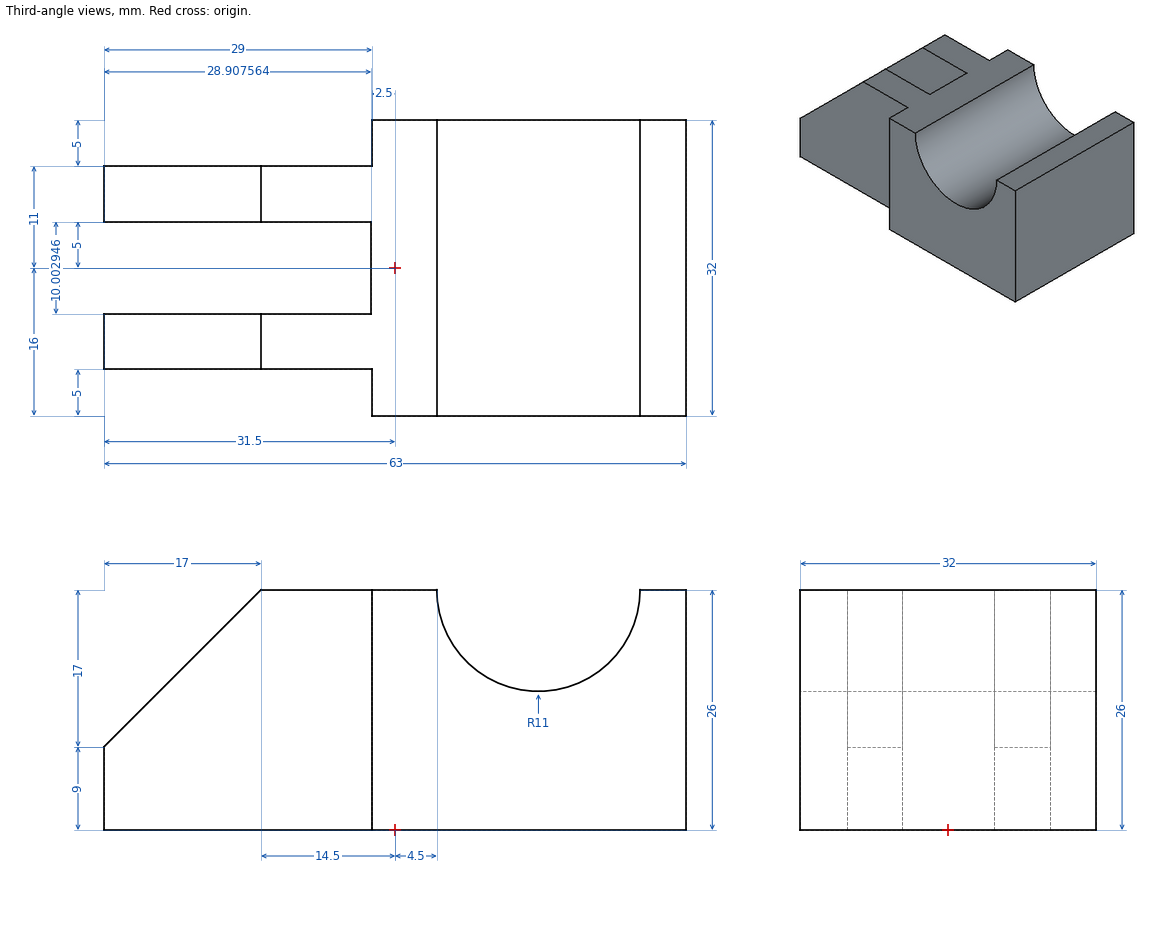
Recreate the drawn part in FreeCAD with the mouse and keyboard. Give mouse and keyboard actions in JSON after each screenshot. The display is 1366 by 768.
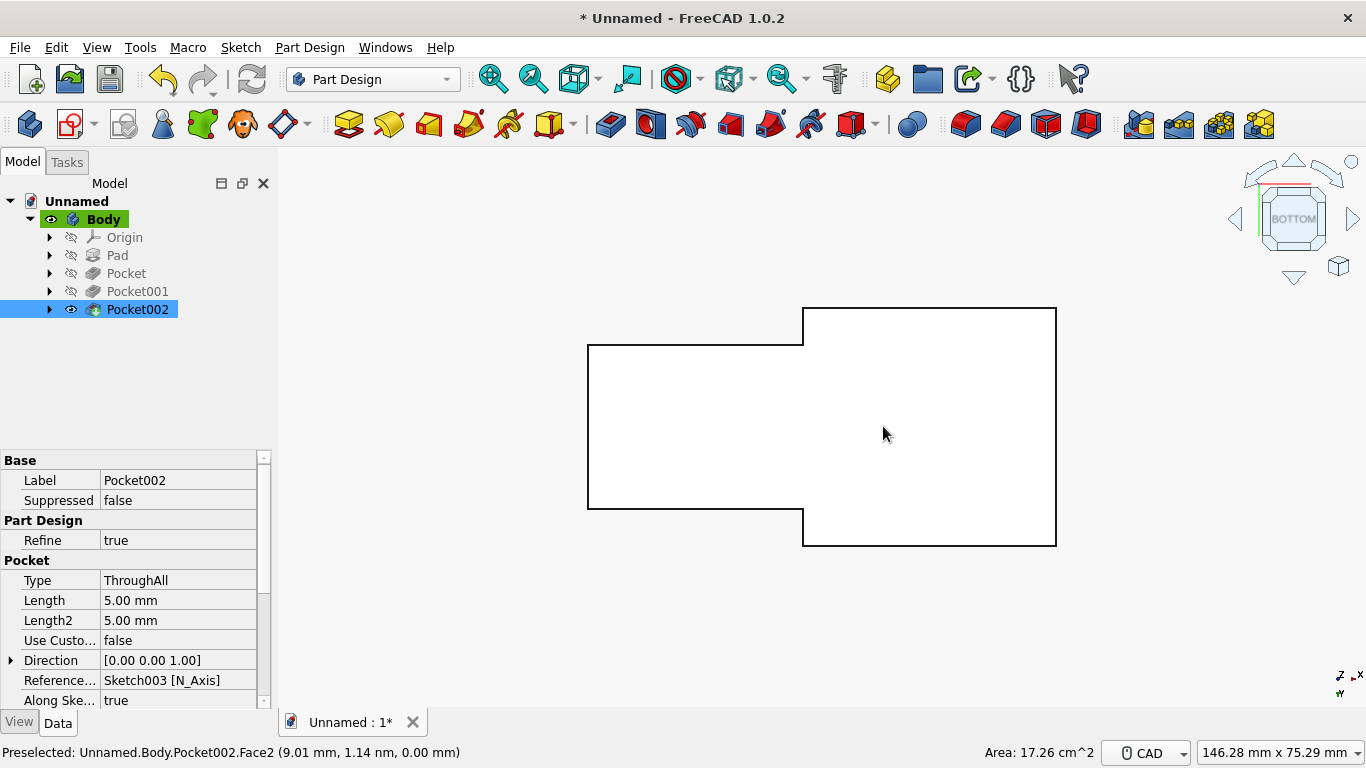
{"action": "left_click", "coordinate": [70, 124]}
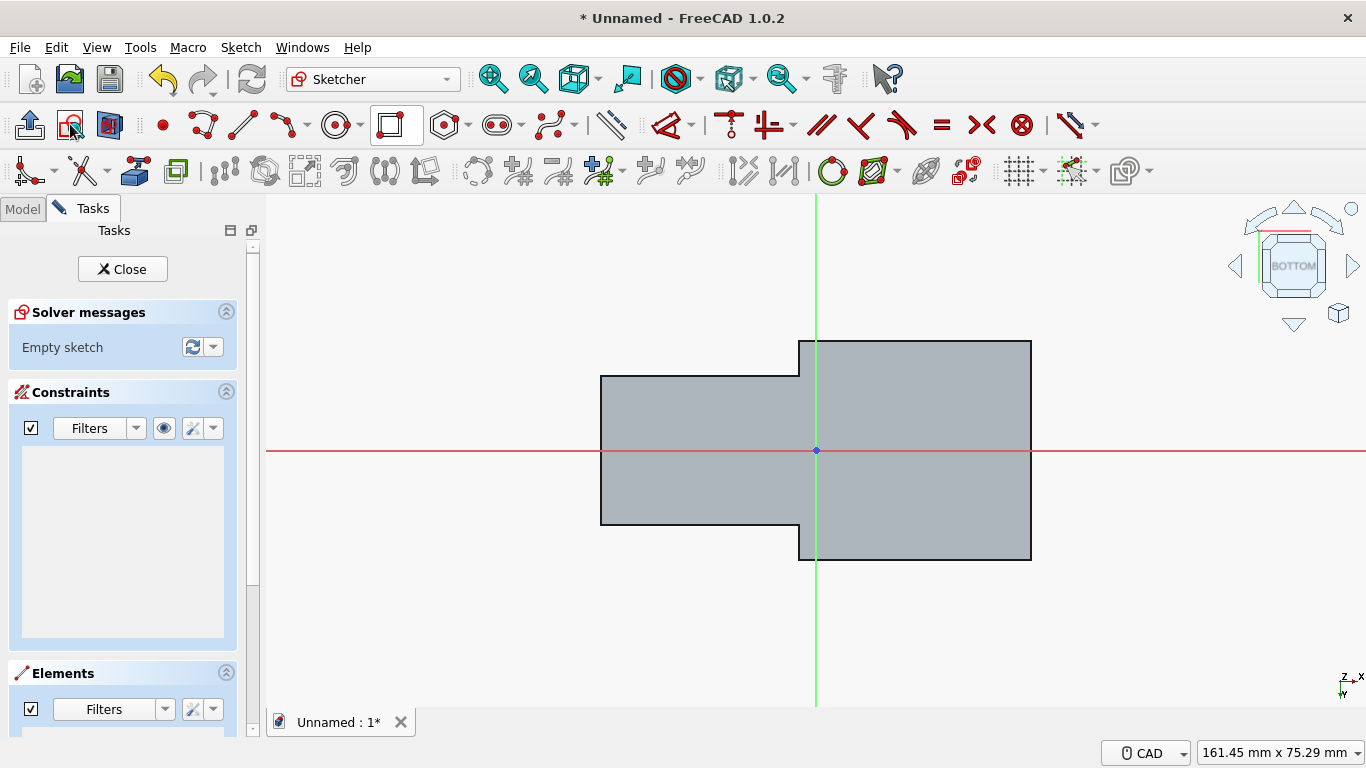
{"action": "scroll", "coordinate": [686, 450], "scroll_direction": "up", "scroll_amount": 5}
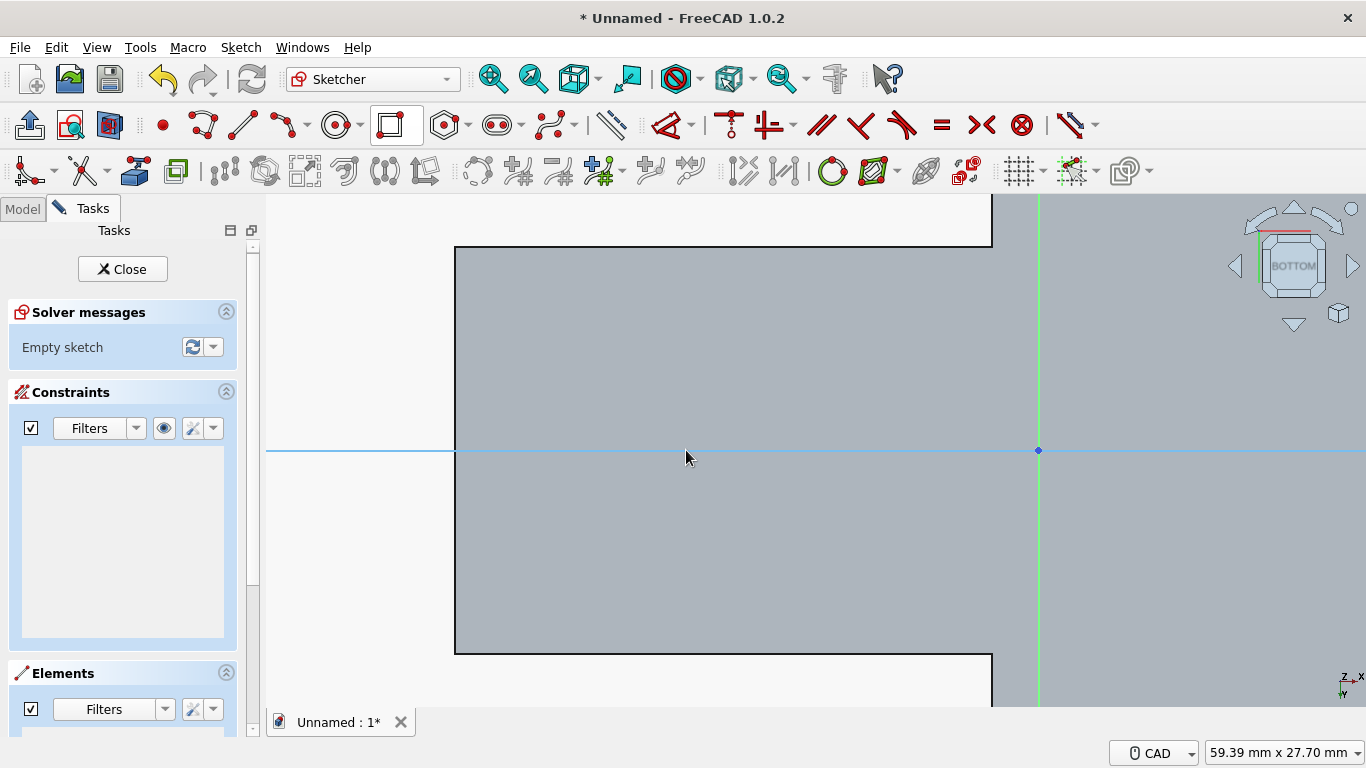
{"action": "left_click", "coordinate": [390, 126]}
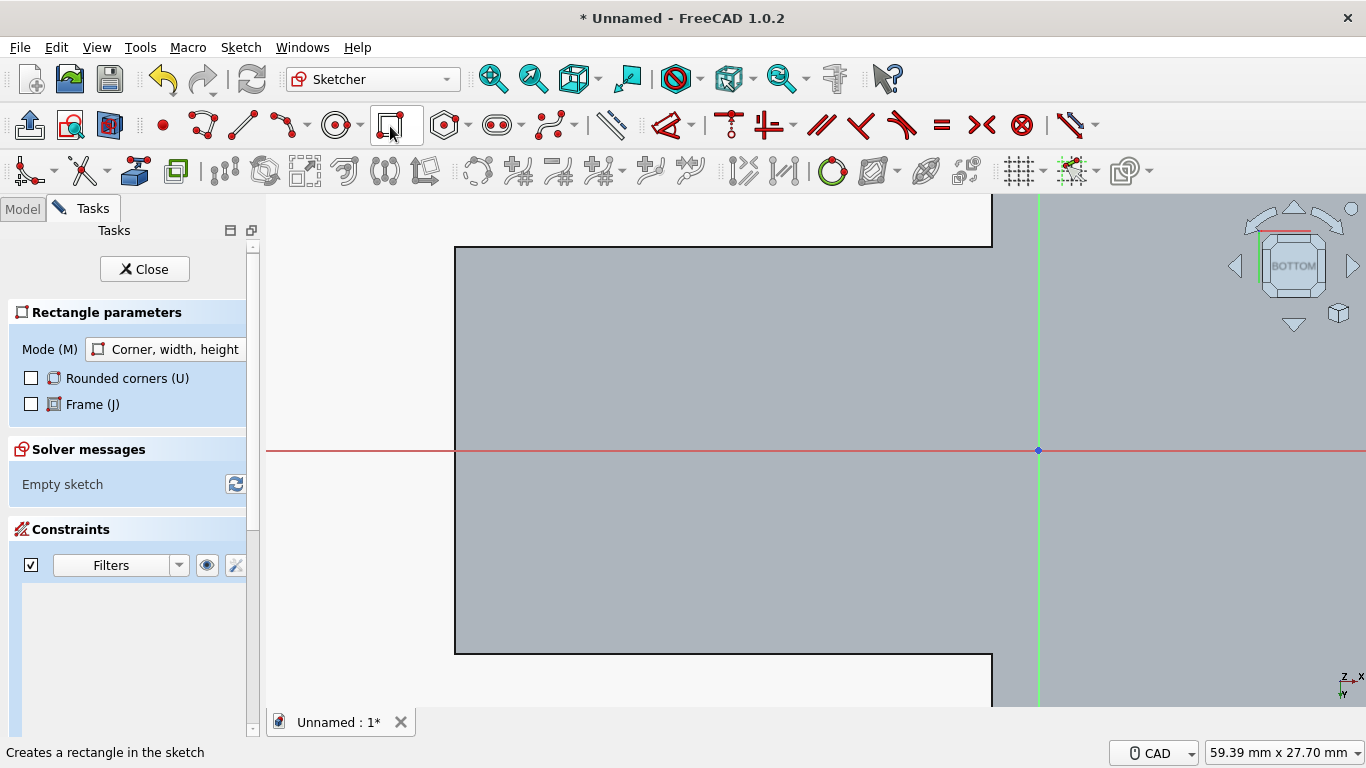
{"action": "left_click", "coordinate": [455, 358]}
{"action": "left_click", "coordinate": [991, 543]}
{"action": "key", "text": "Escape"}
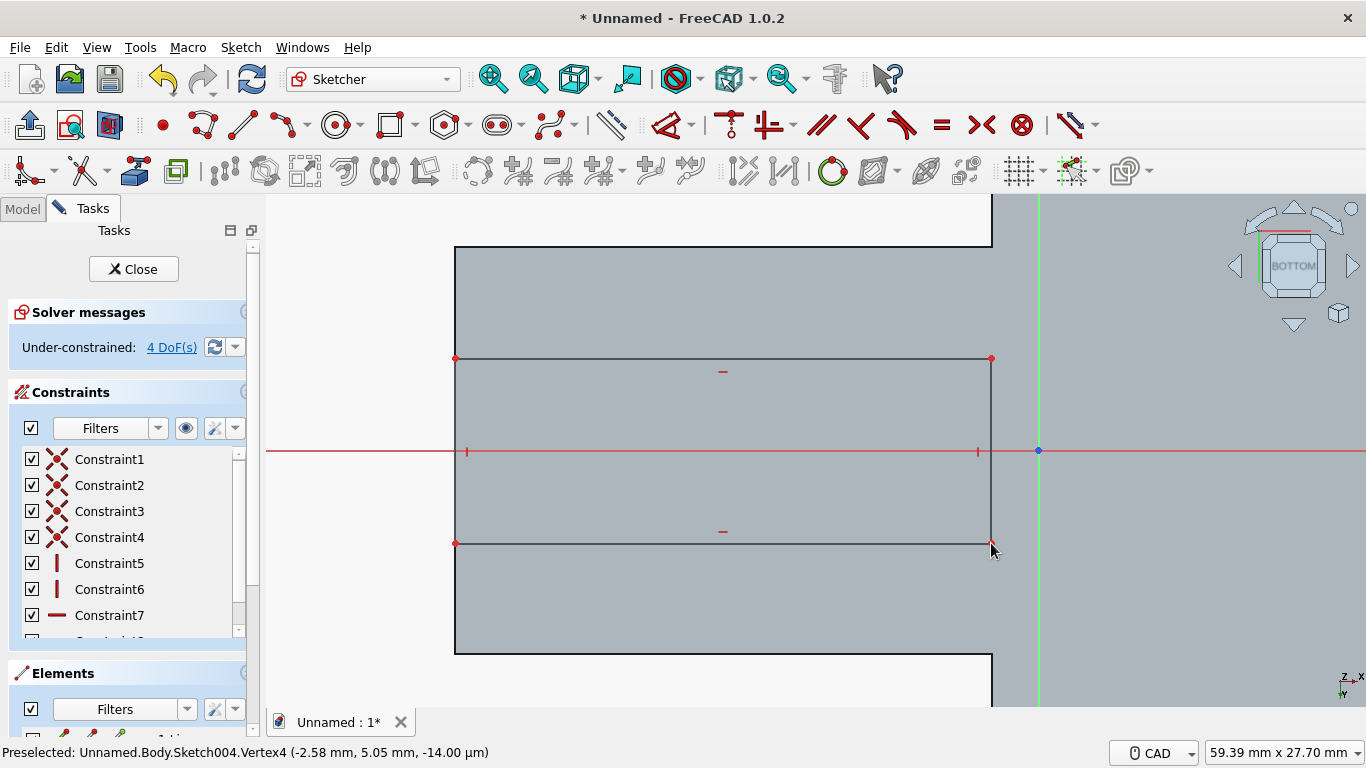
{"action": "left_click", "coordinate": [666, 126]}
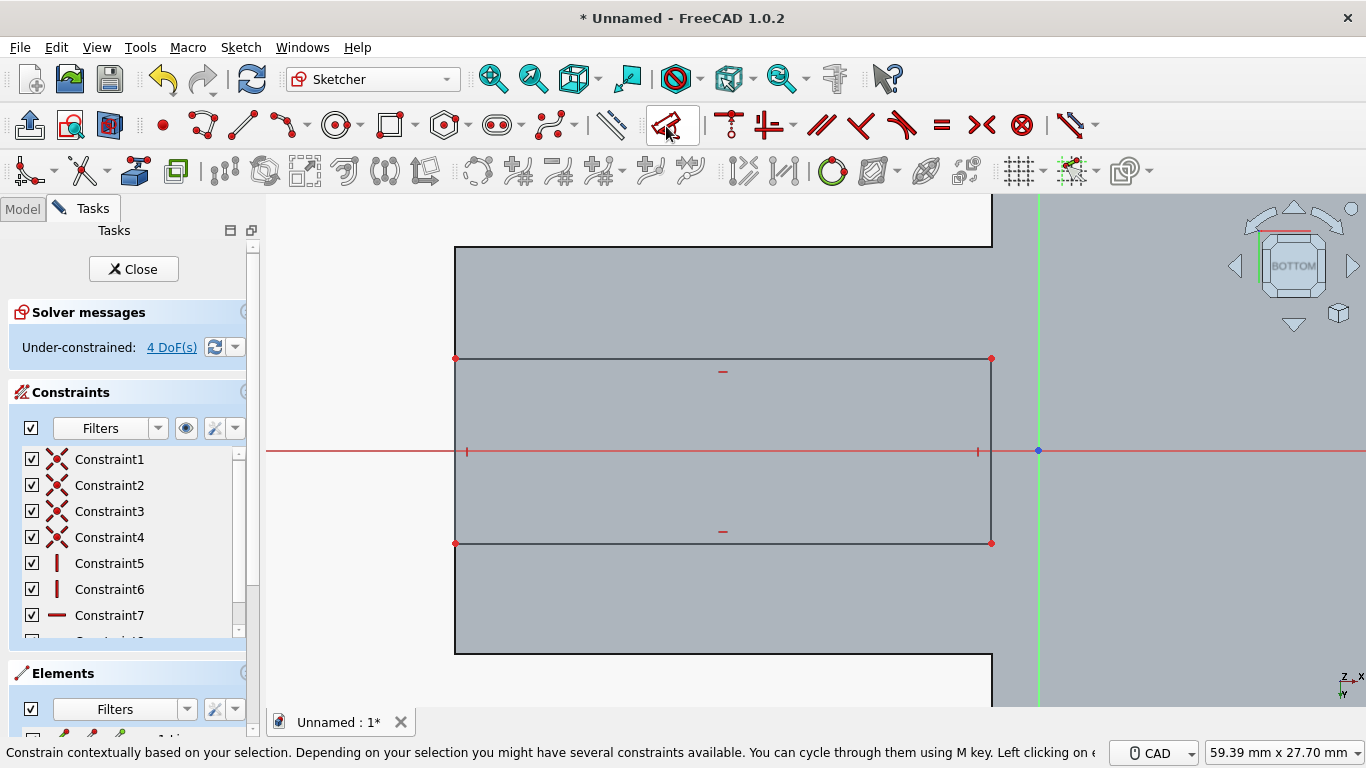
{"action": "left_click", "coordinate": [455, 544]}
{"action": "left_click", "coordinate": [421, 497]}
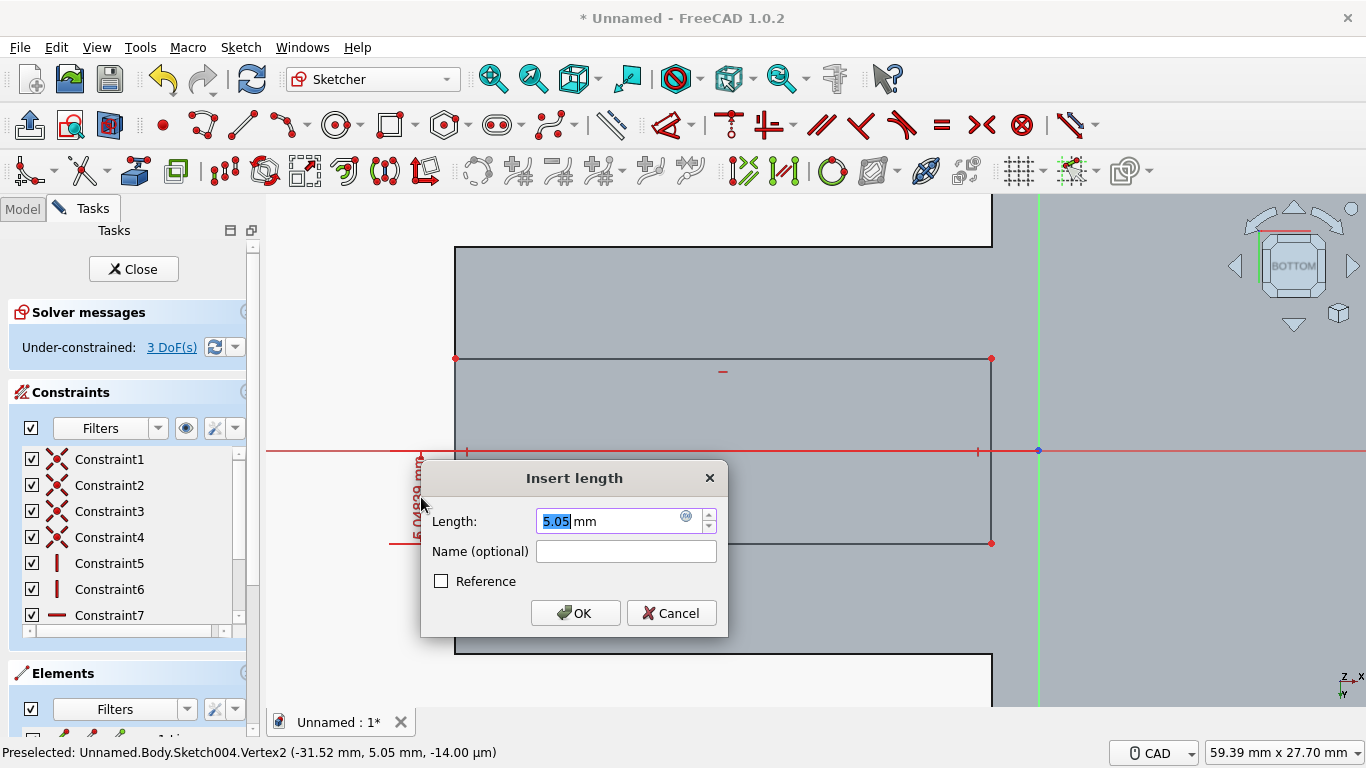
{"action": "type", "text": "5"}
{"action": "key", "text": "Return"}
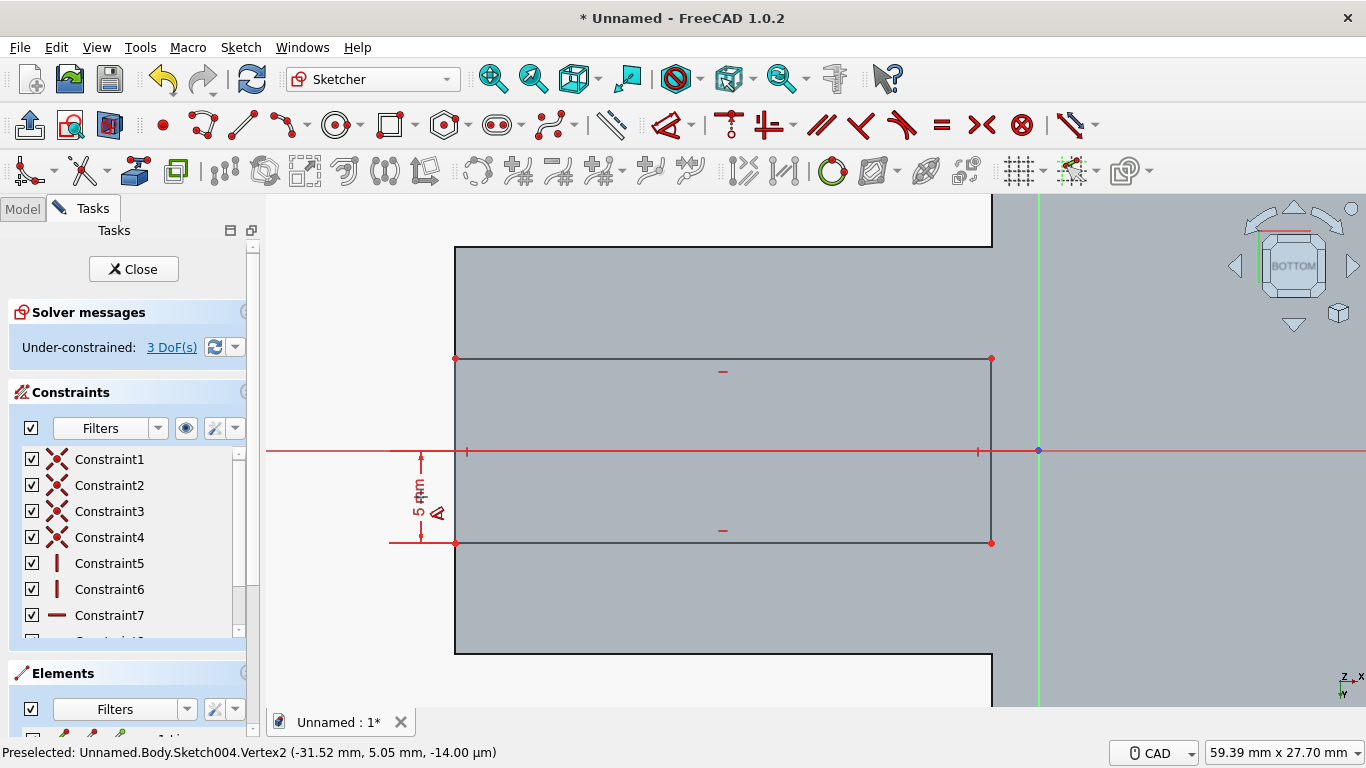
{"action": "left_click", "coordinate": [455, 359]}
{"action": "left_click", "coordinate": [747, 325]}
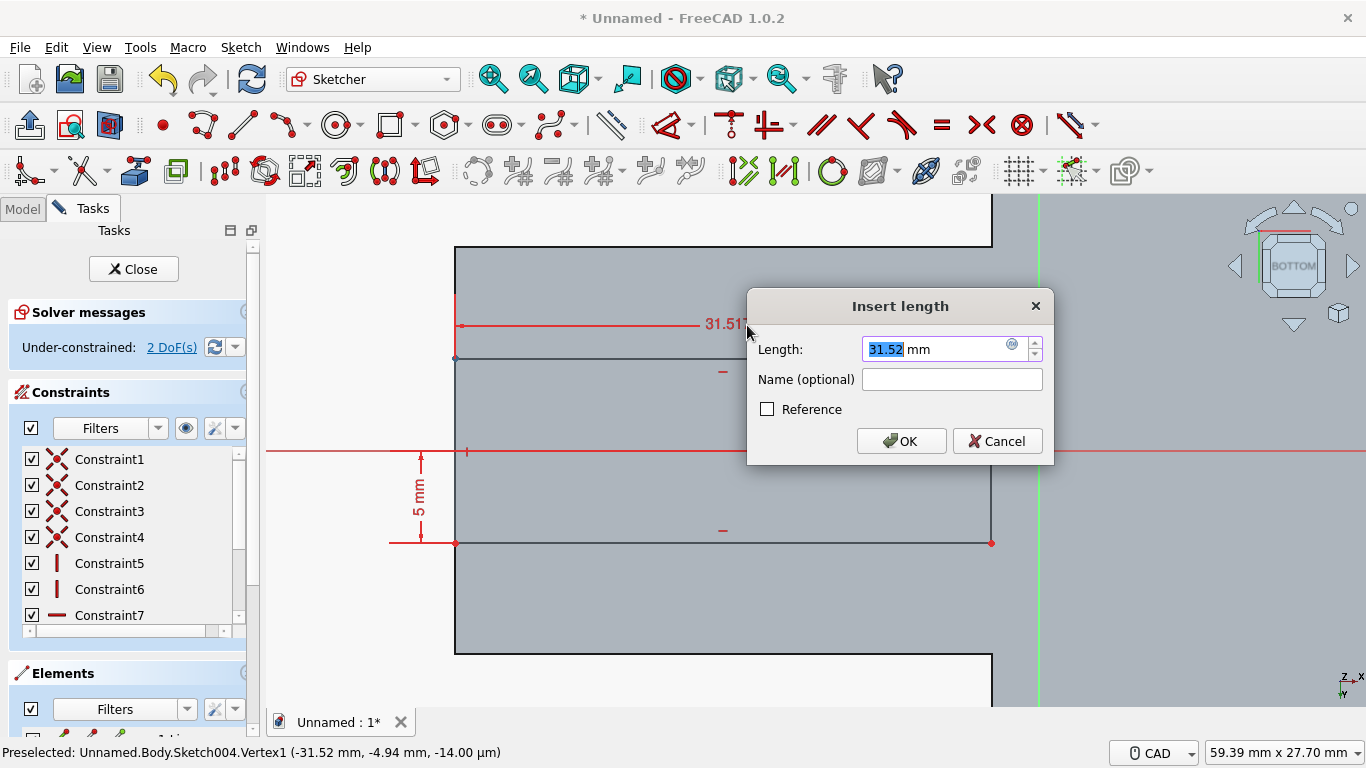
{"action": "type", "text": "31.5"}
{"action": "key", "text": "Return"}